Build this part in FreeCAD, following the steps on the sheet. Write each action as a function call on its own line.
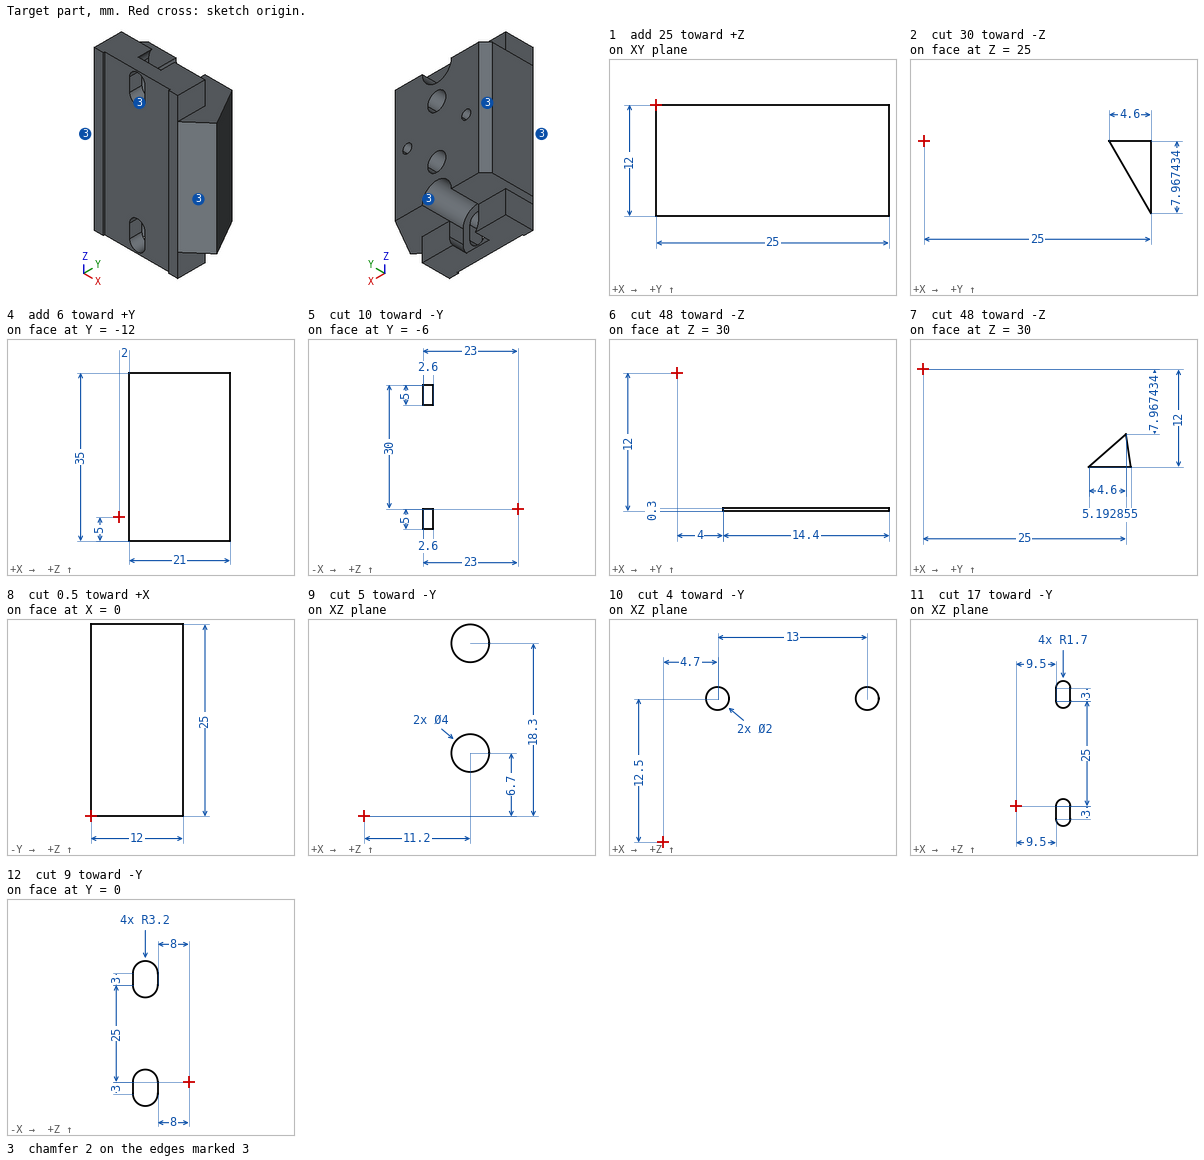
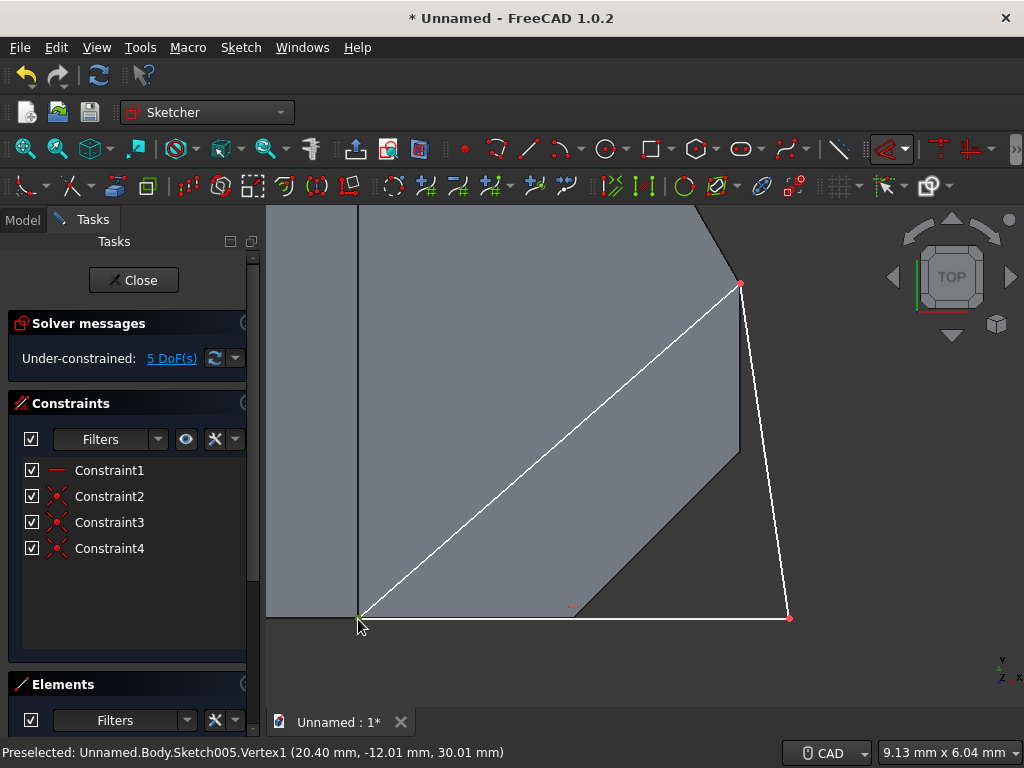
click(908, 150)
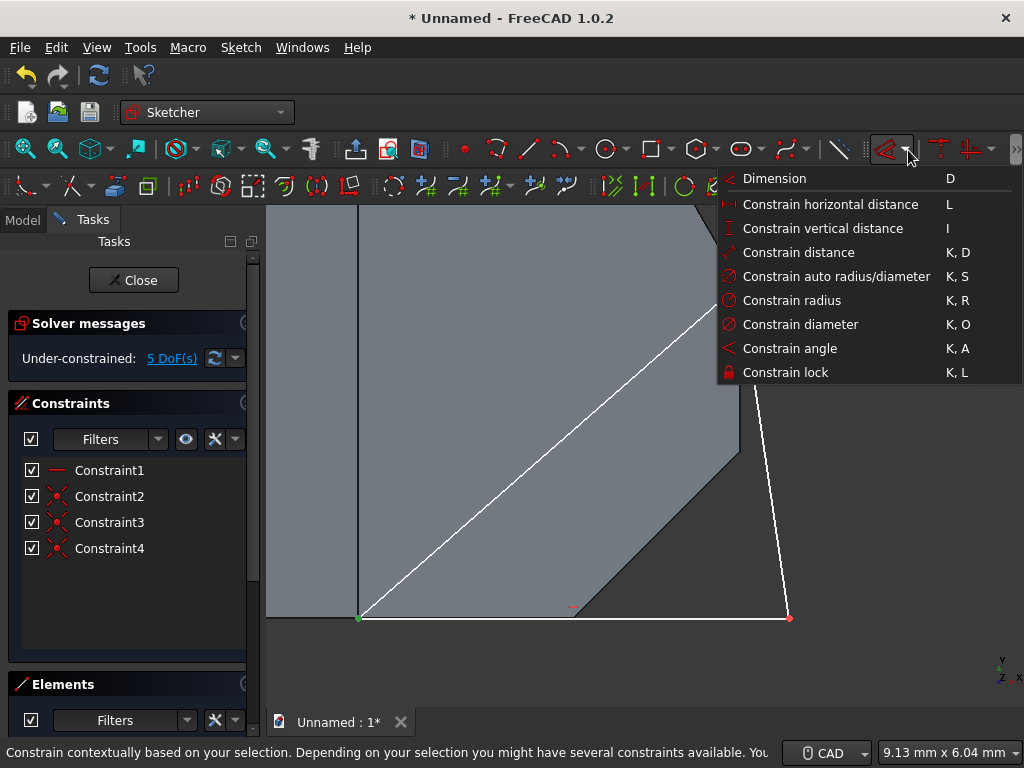
click(870, 228)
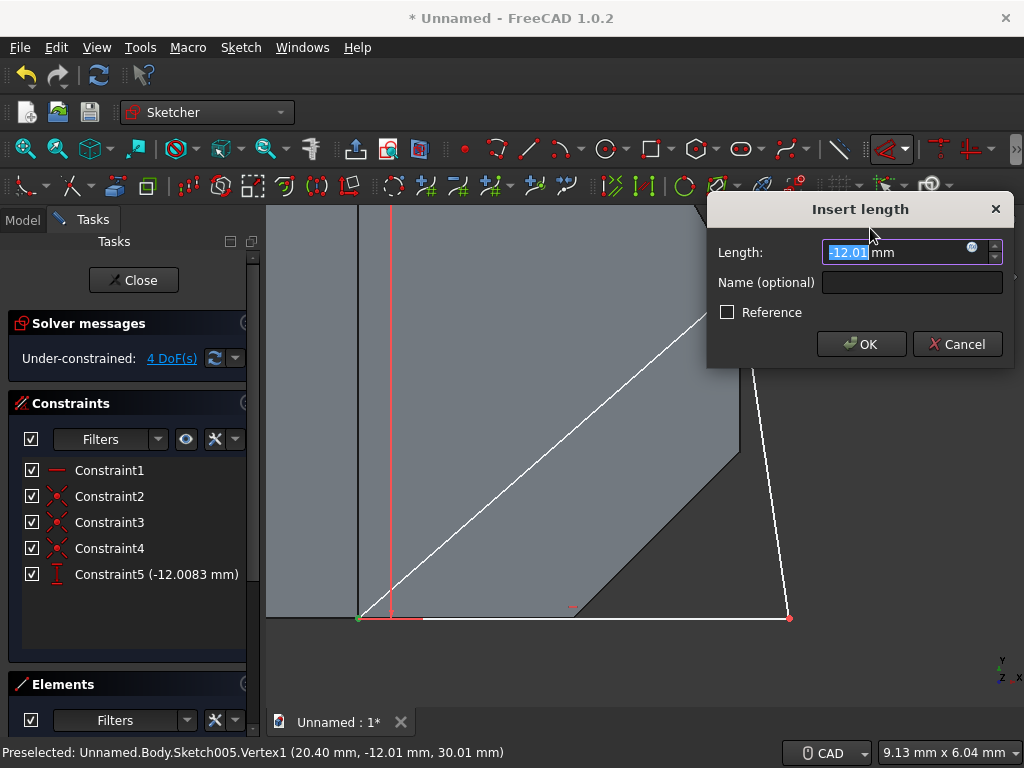
text(-12)
key(Return)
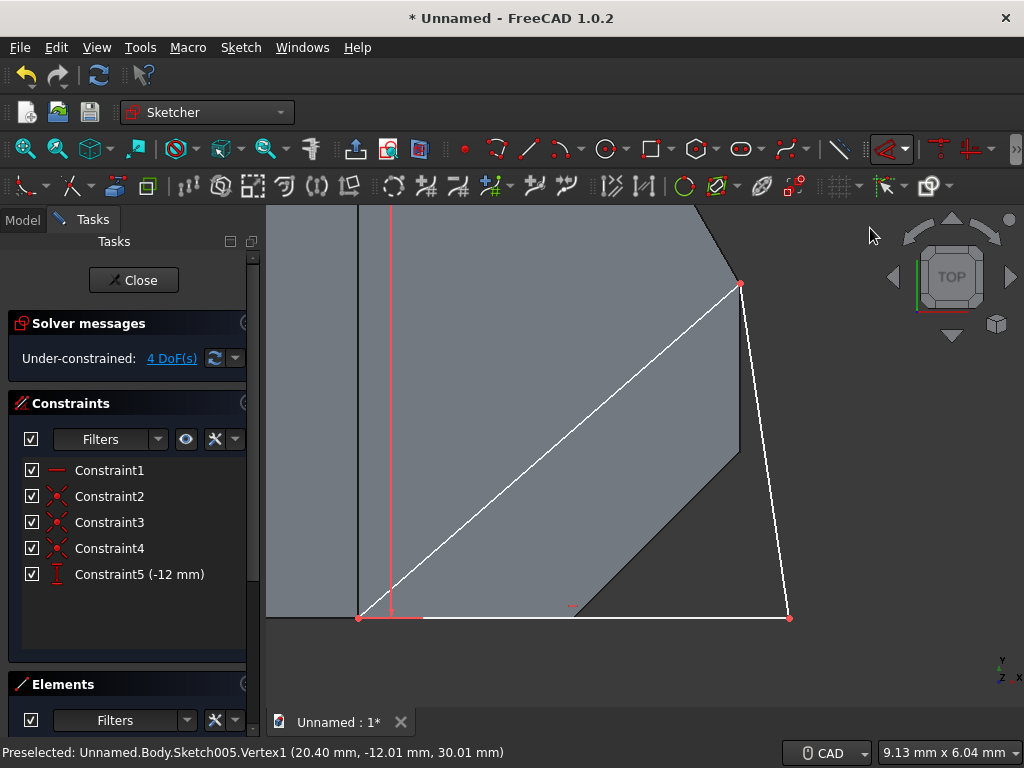
click(740, 284)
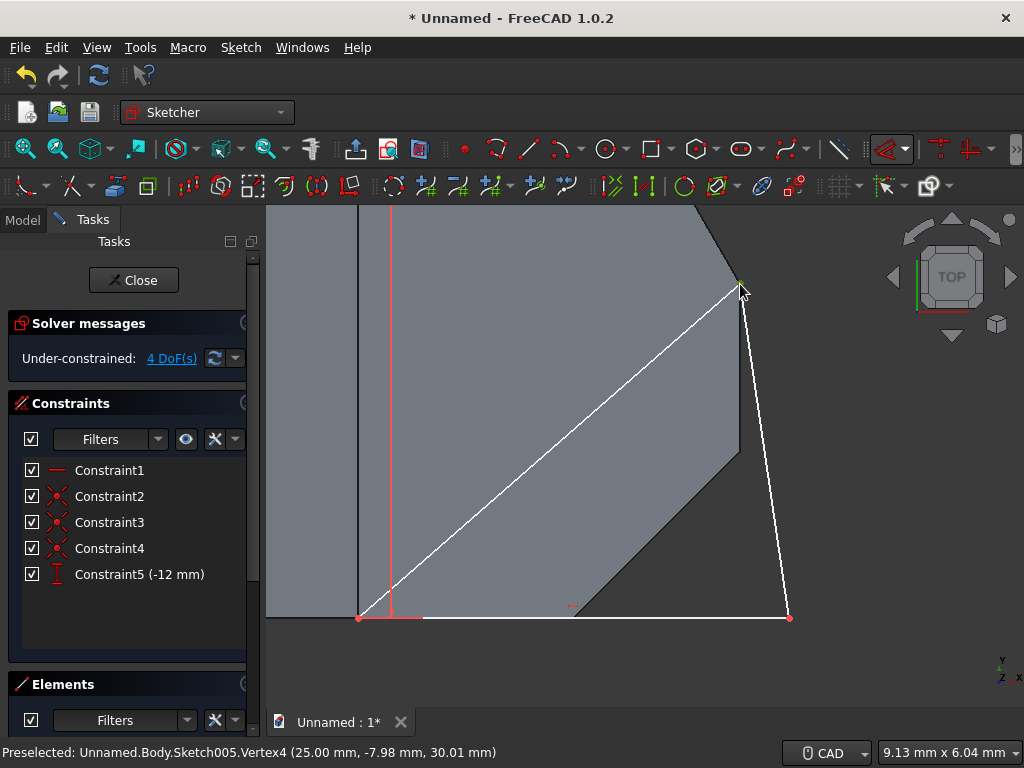
key(l)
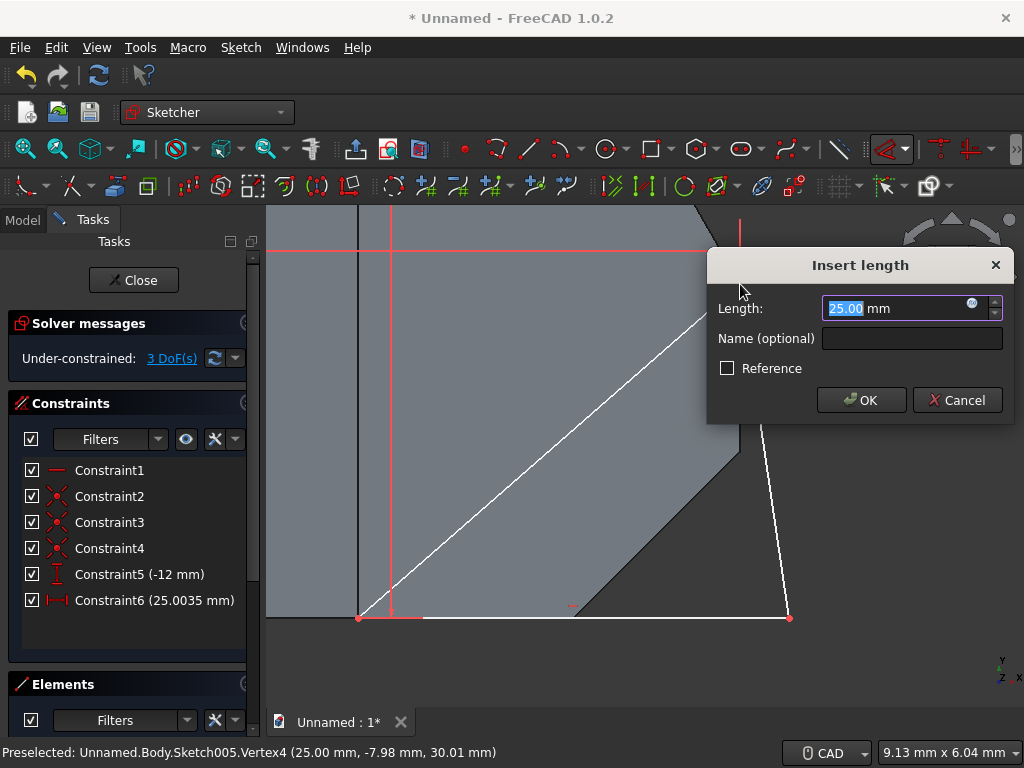
text(25)
key(Return)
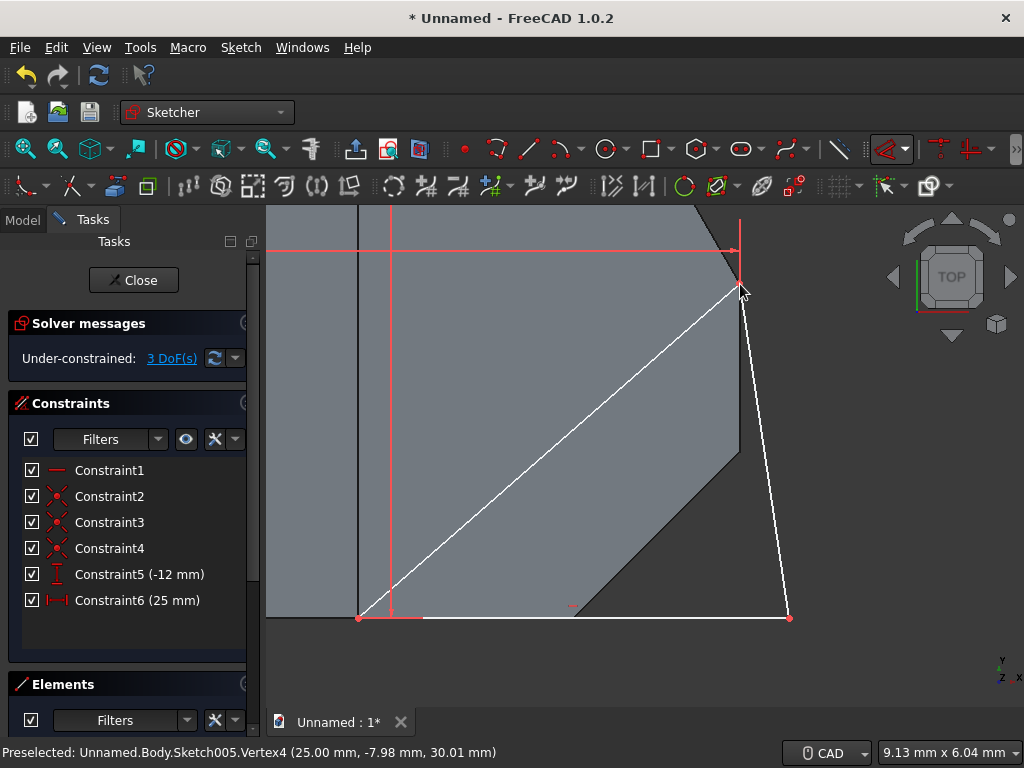
click(625, 384)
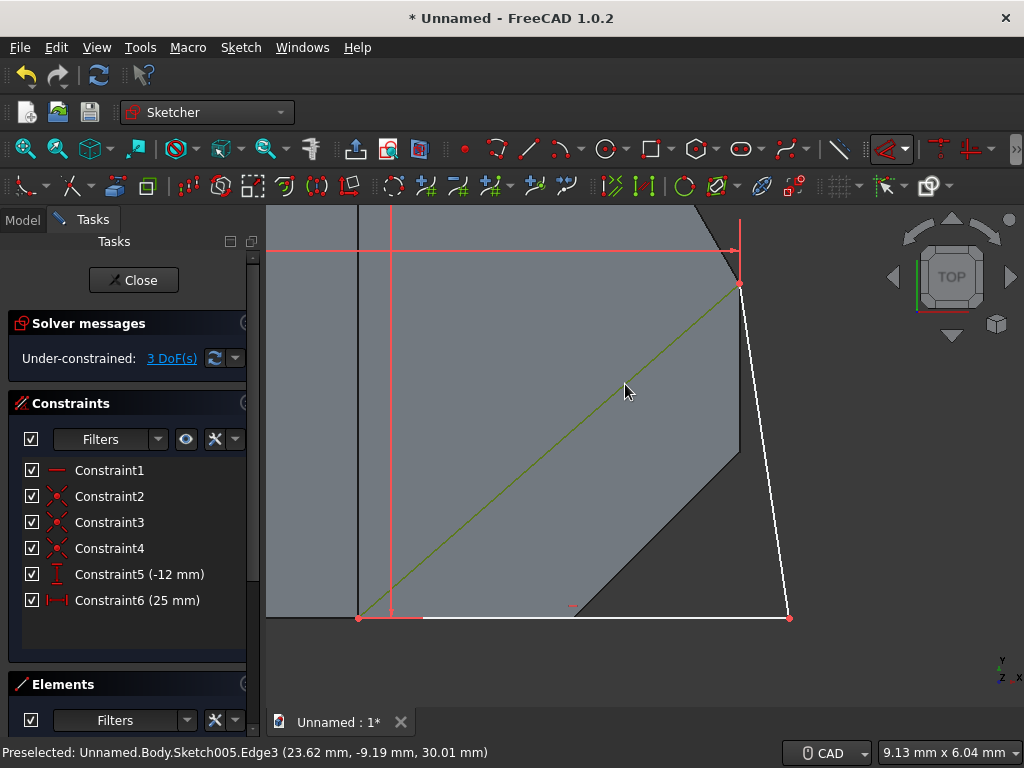
click(908, 150)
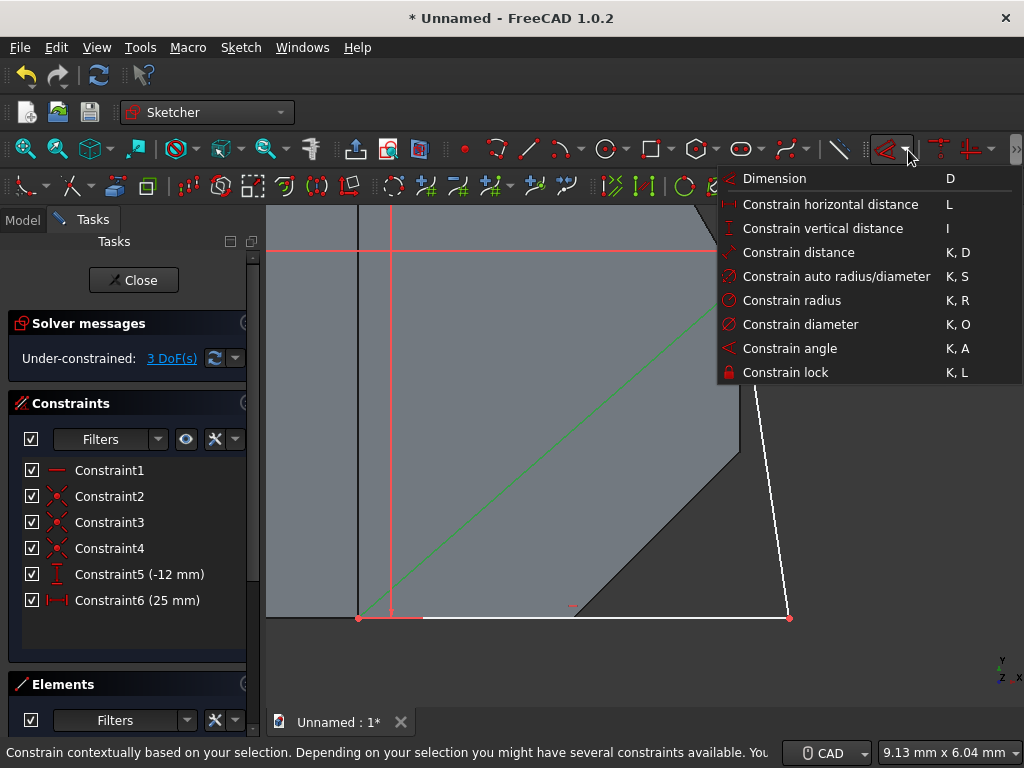
click(870, 204)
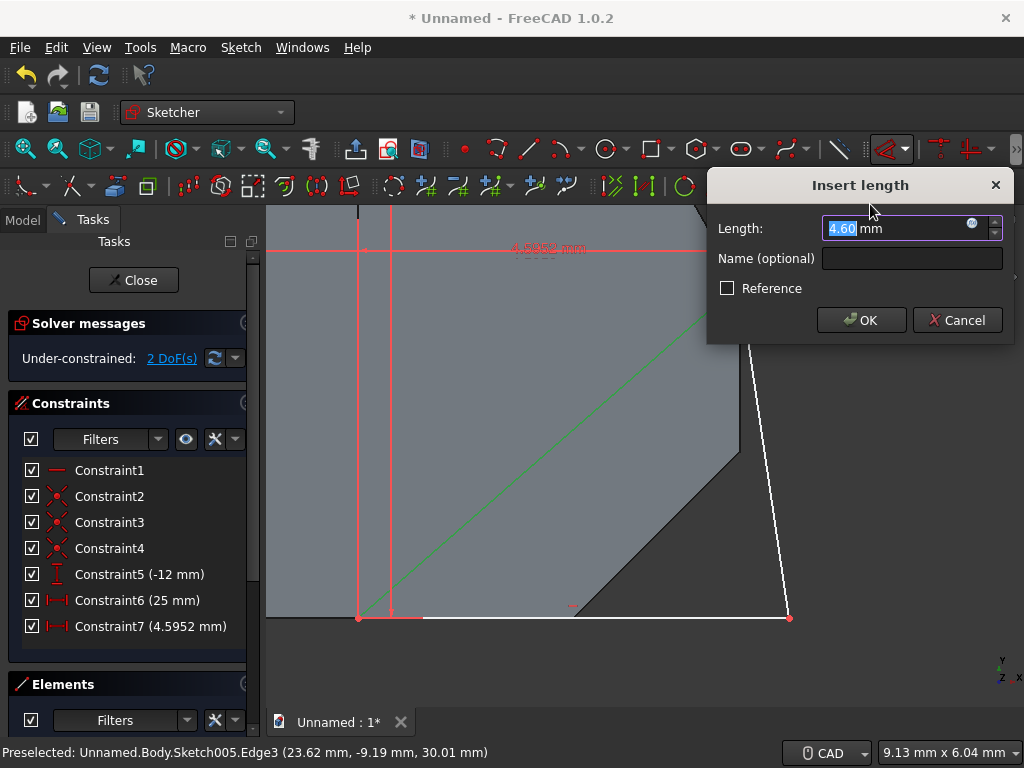
text(4.6)
key(Return)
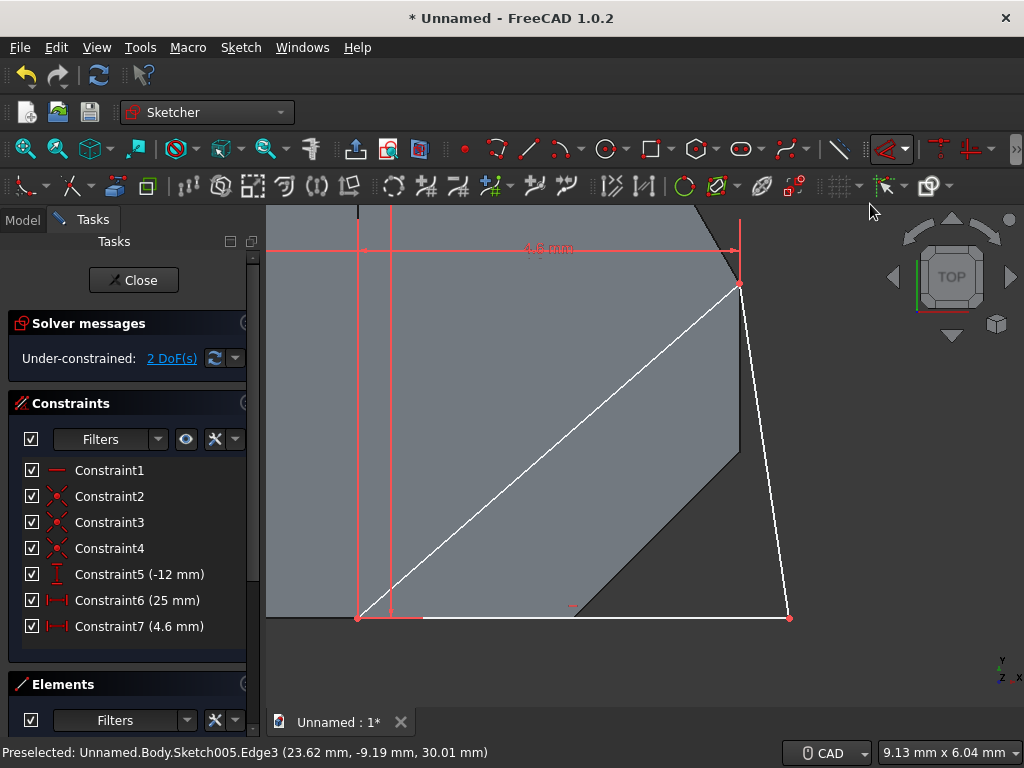
click(487, 618)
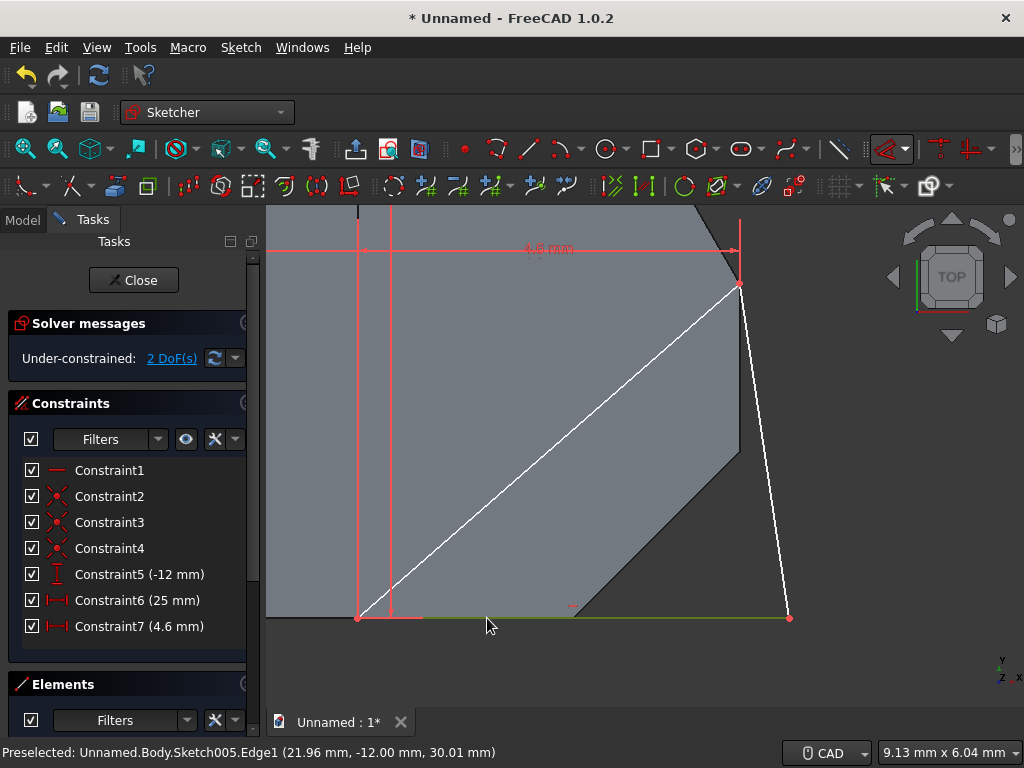
key(l)